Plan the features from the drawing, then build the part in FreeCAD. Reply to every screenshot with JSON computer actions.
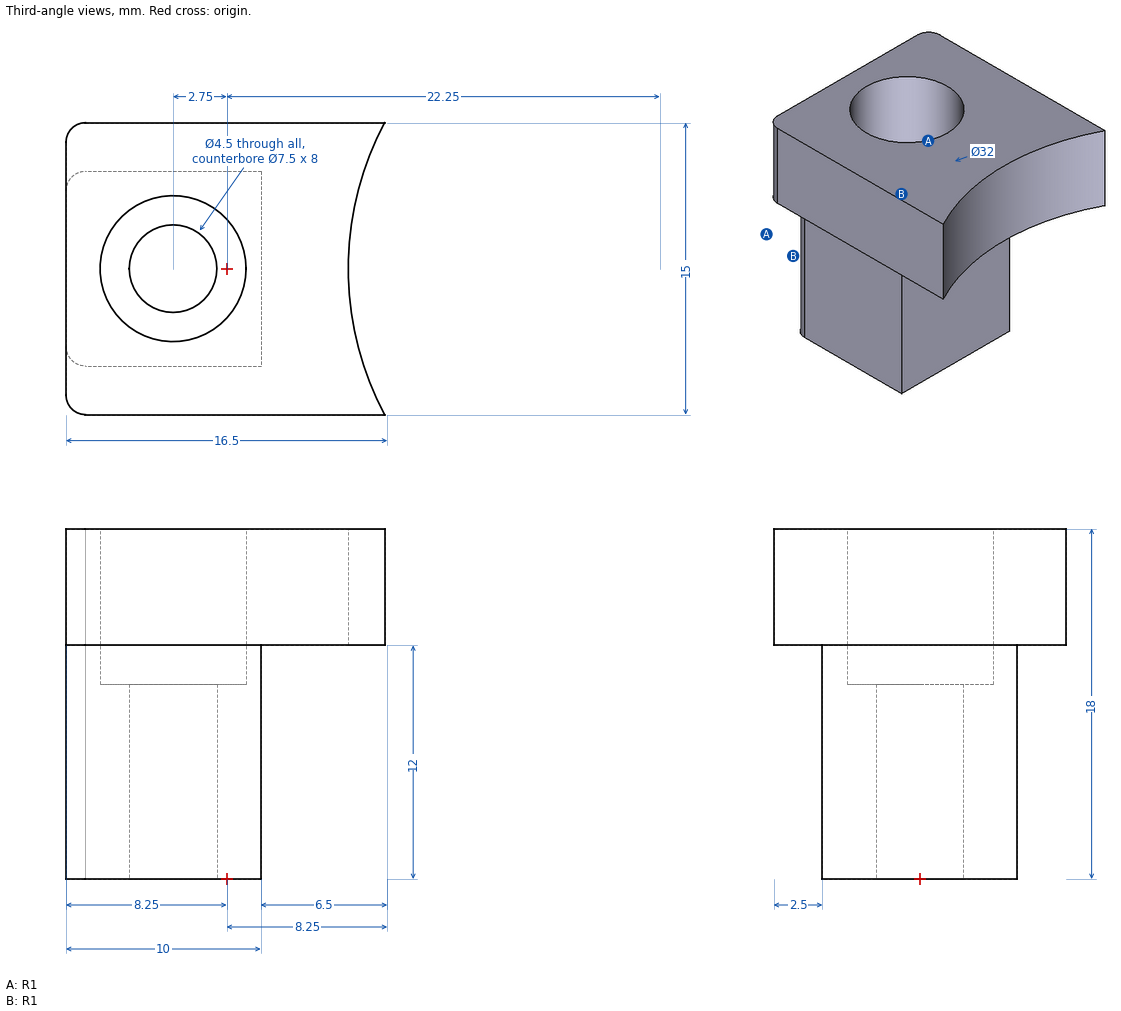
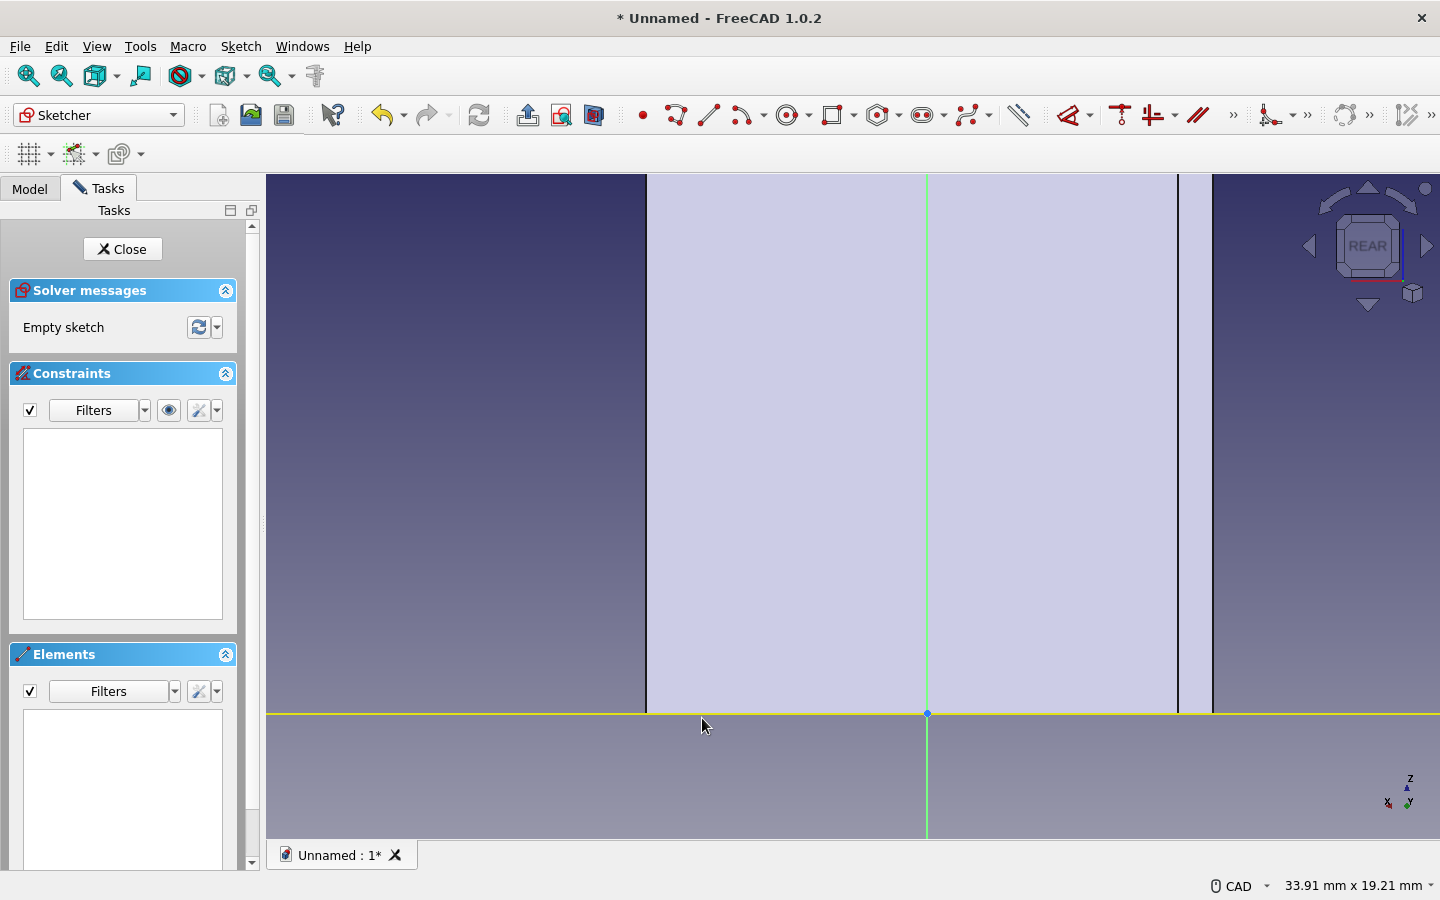
{"action": "key", "text": "g r"}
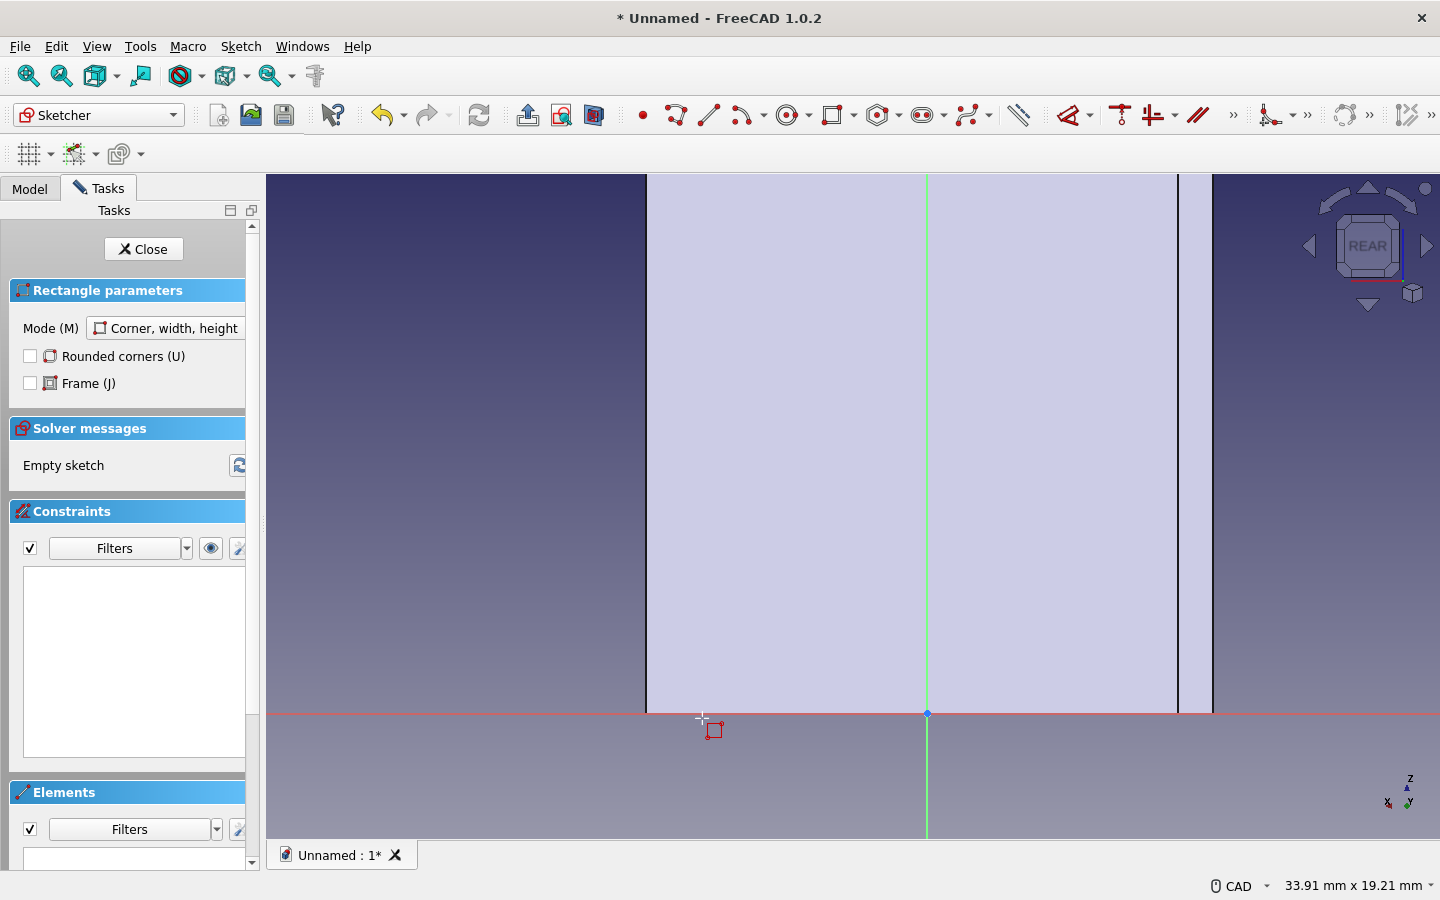
{"action": "left_click", "coordinate": [641, 298]}
{"action": "left_click", "coordinate": [867, 714]}
{"action": "key", "text": "Escape"}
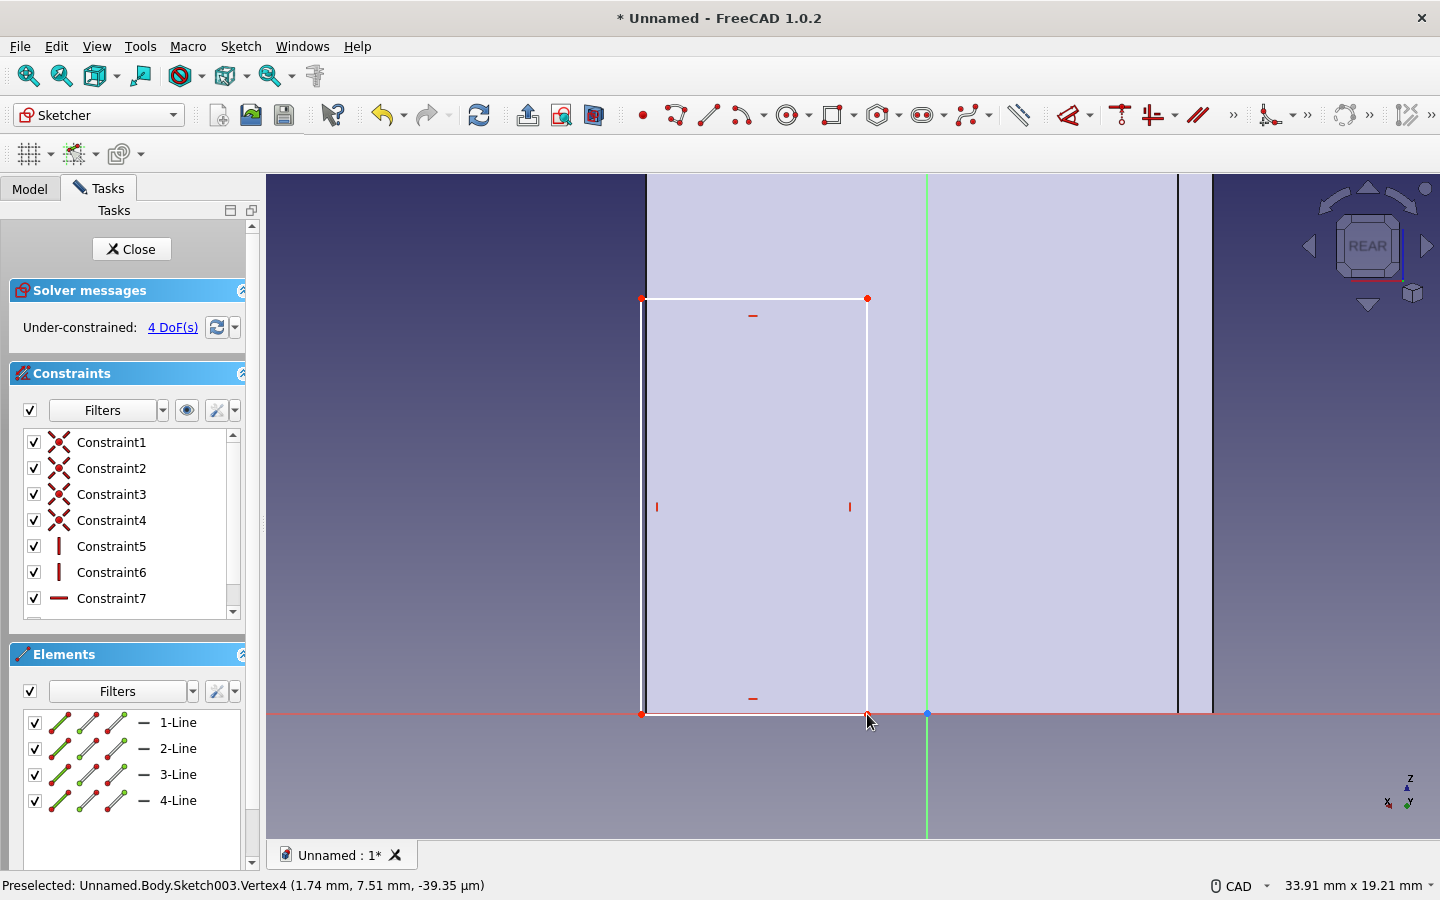
{"action": "left_click", "coordinate": [641, 715]}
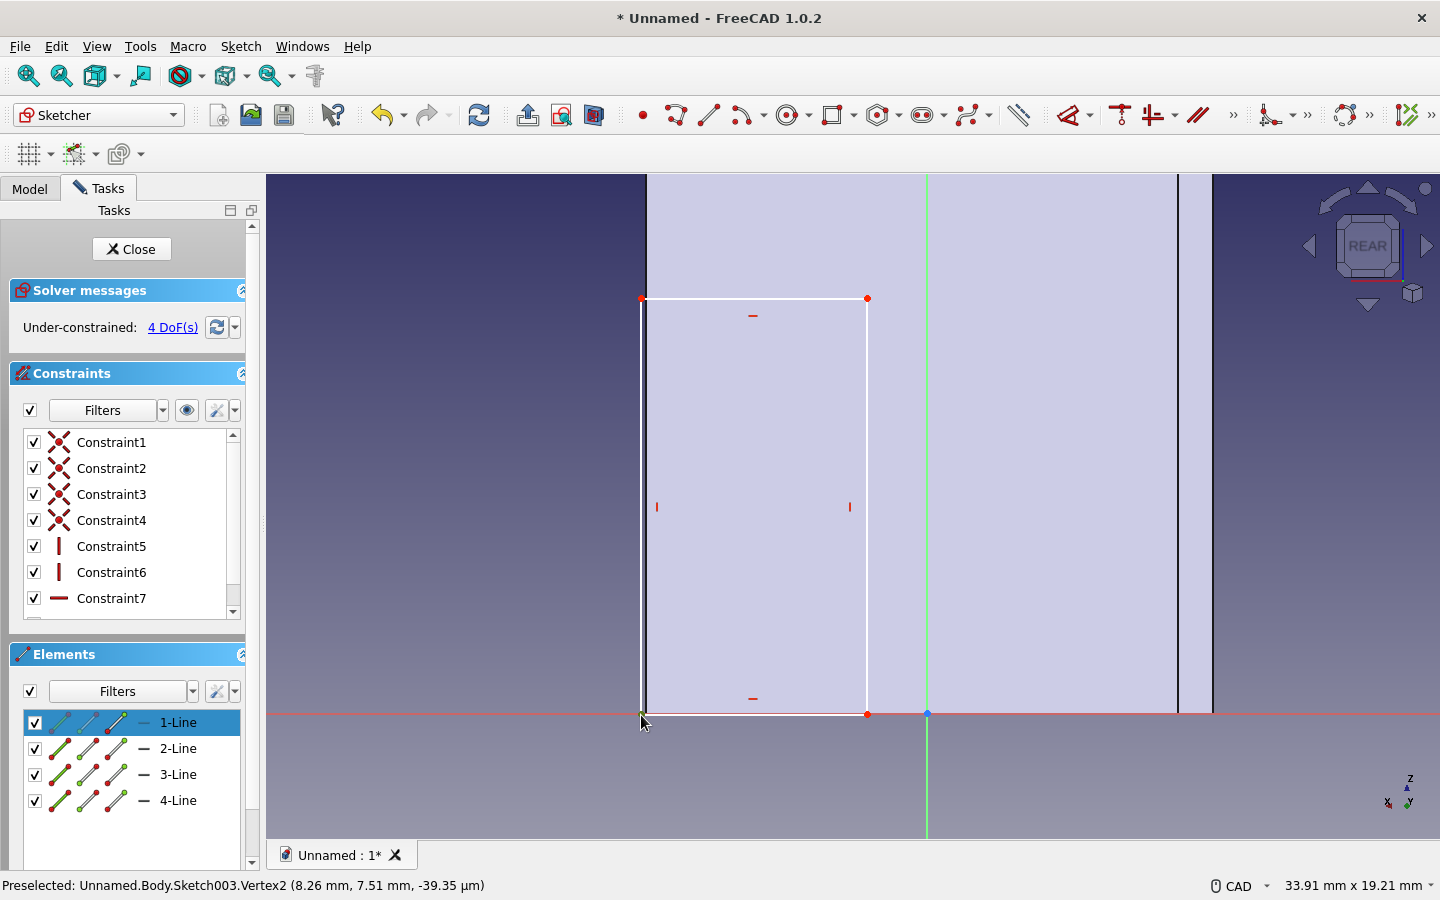
{"action": "left_click", "coordinate": [364, 714]}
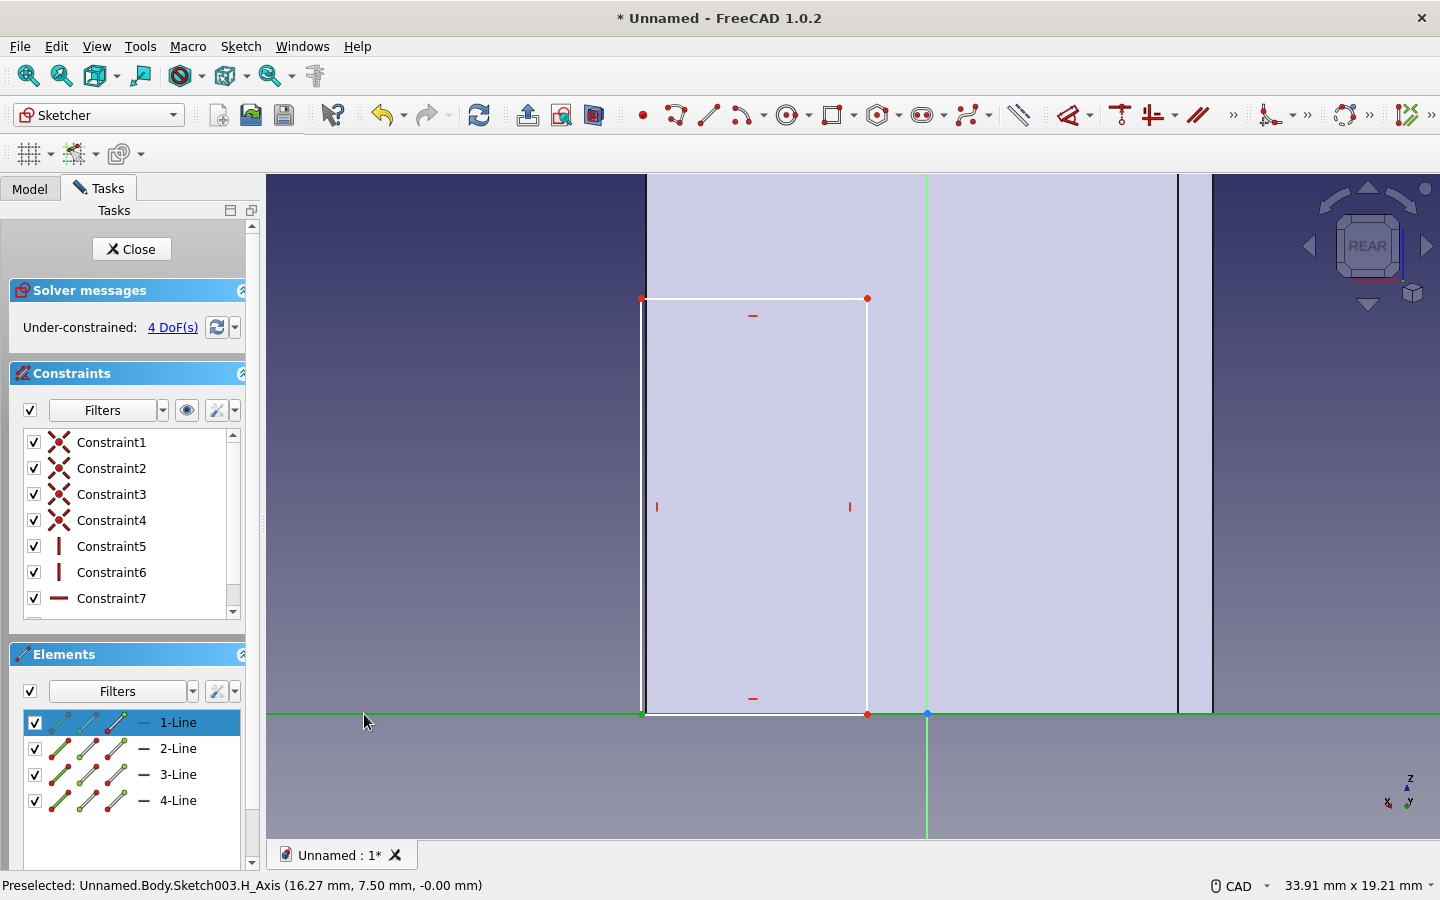
{"action": "key", "text": "c"}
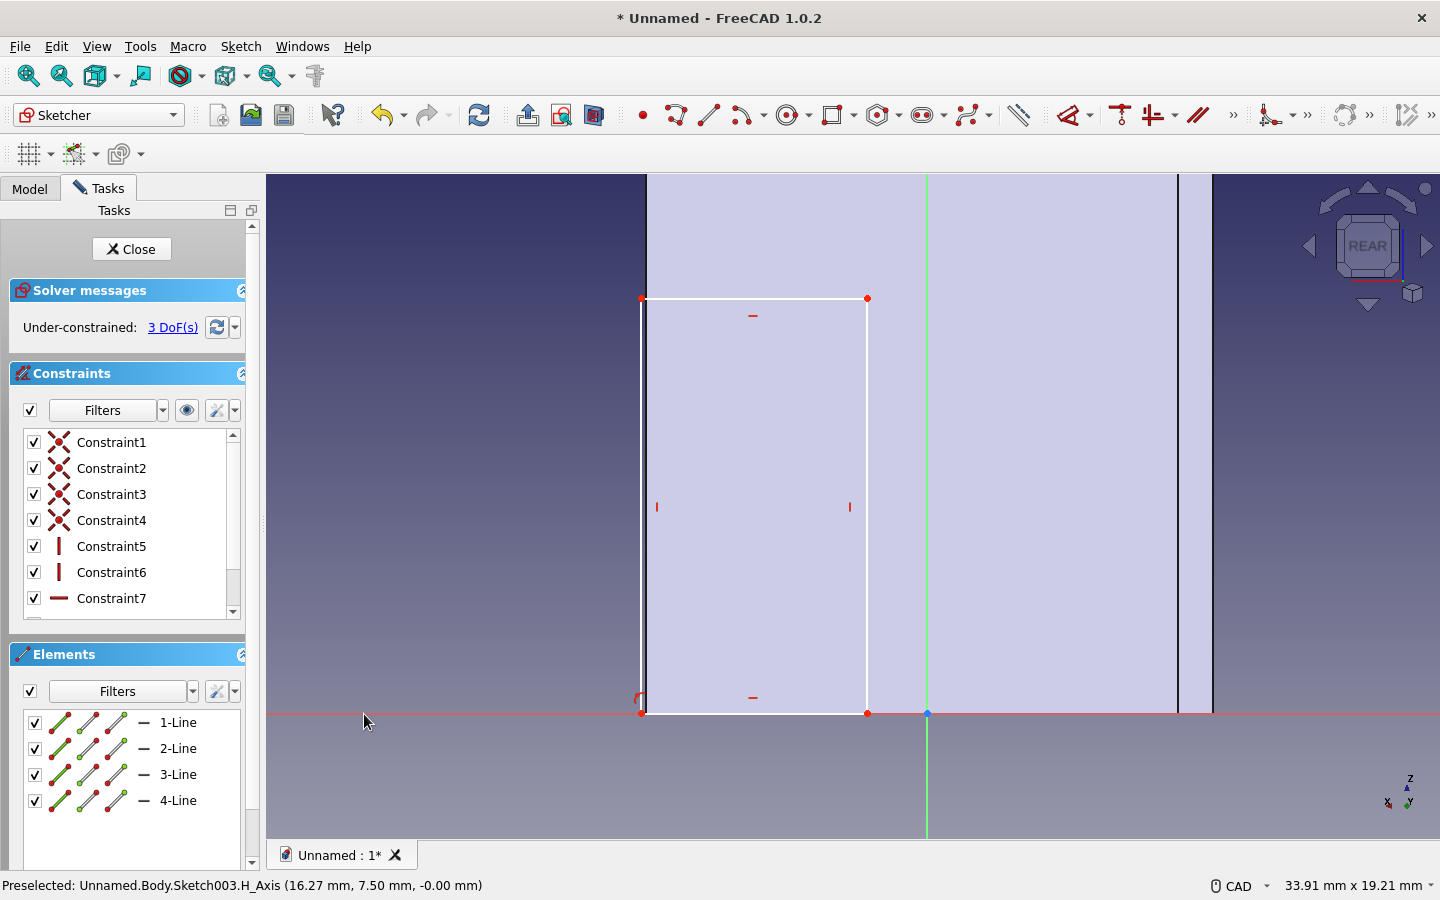
{"action": "key", "text": "d"}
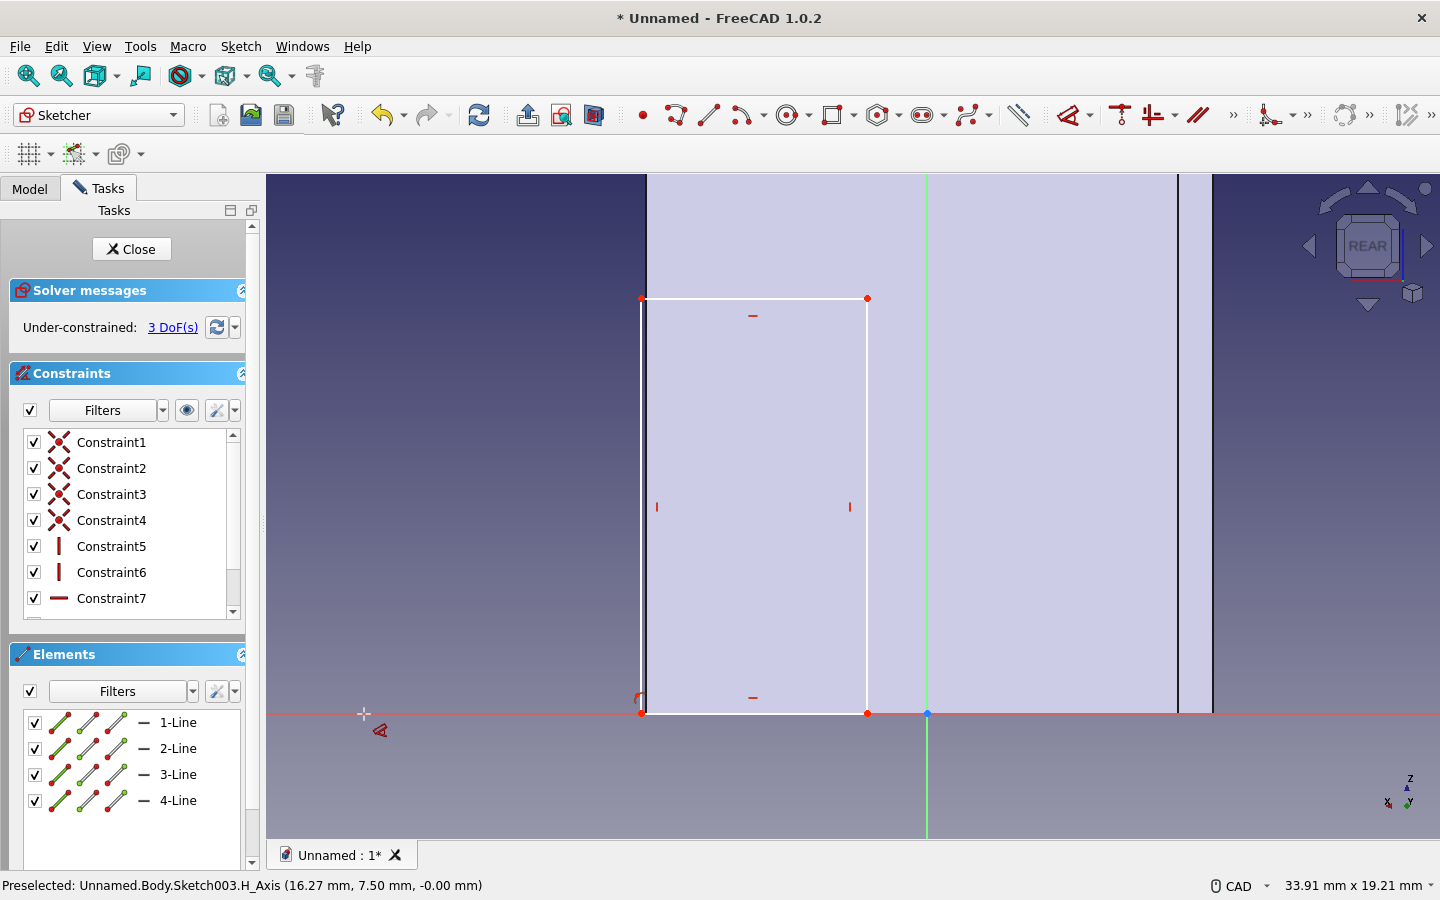
{"action": "left_click", "coordinate": [641, 423]}
{"action": "left_click", "coordinate": [607, 506]}